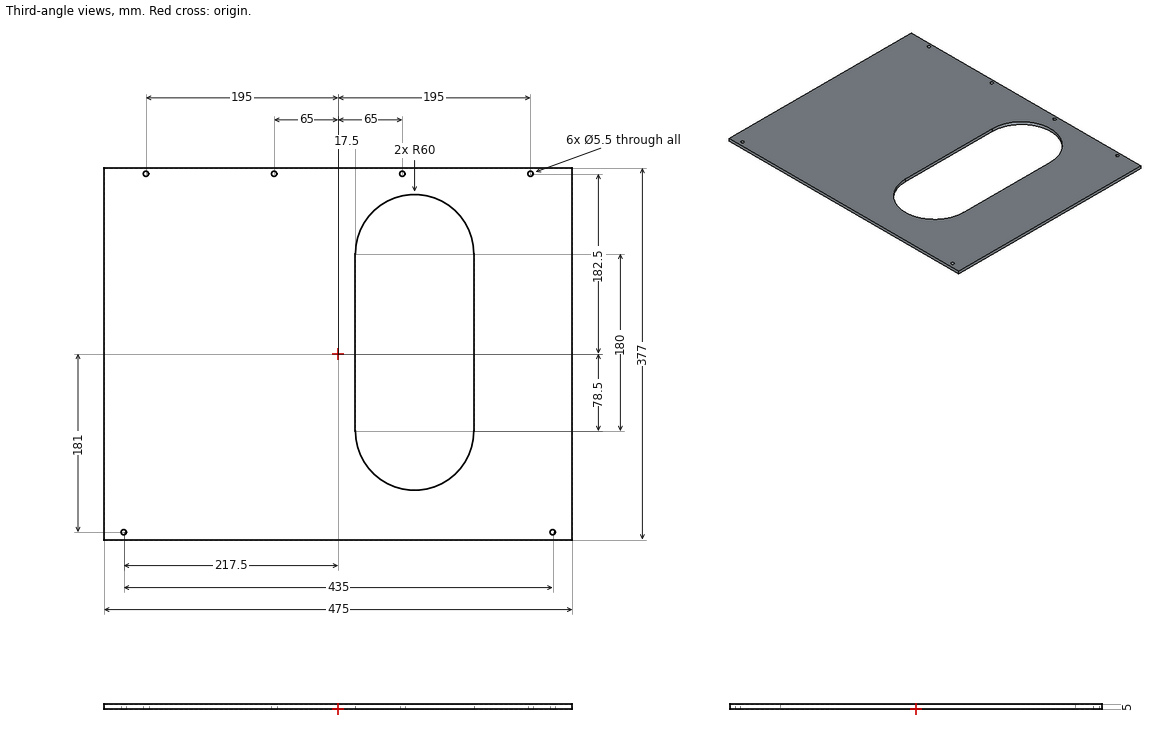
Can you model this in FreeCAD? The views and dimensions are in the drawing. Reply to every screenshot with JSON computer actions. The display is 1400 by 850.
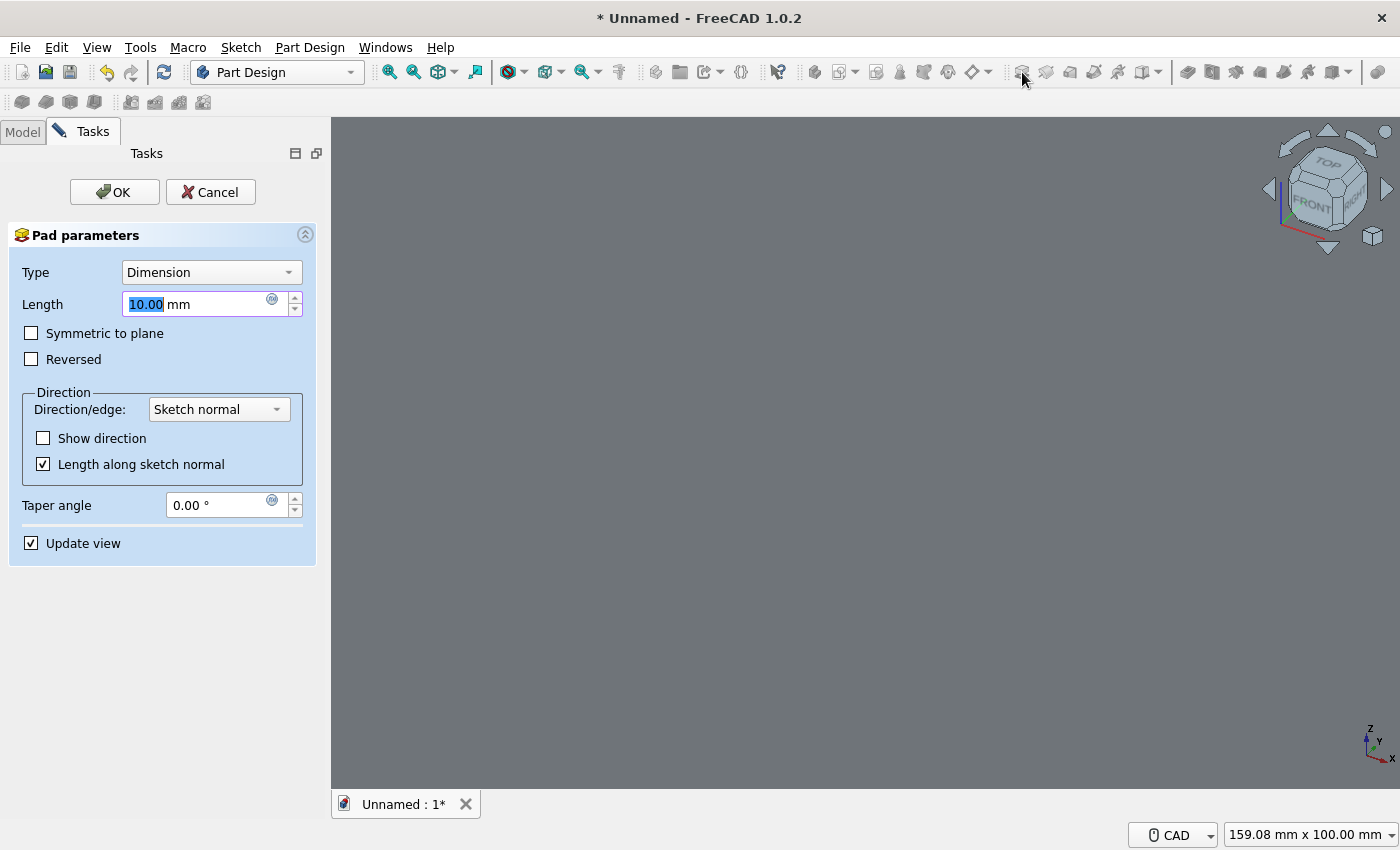
{"action": "type", "text": "5"}
{"action": "key", "text": "Tab"}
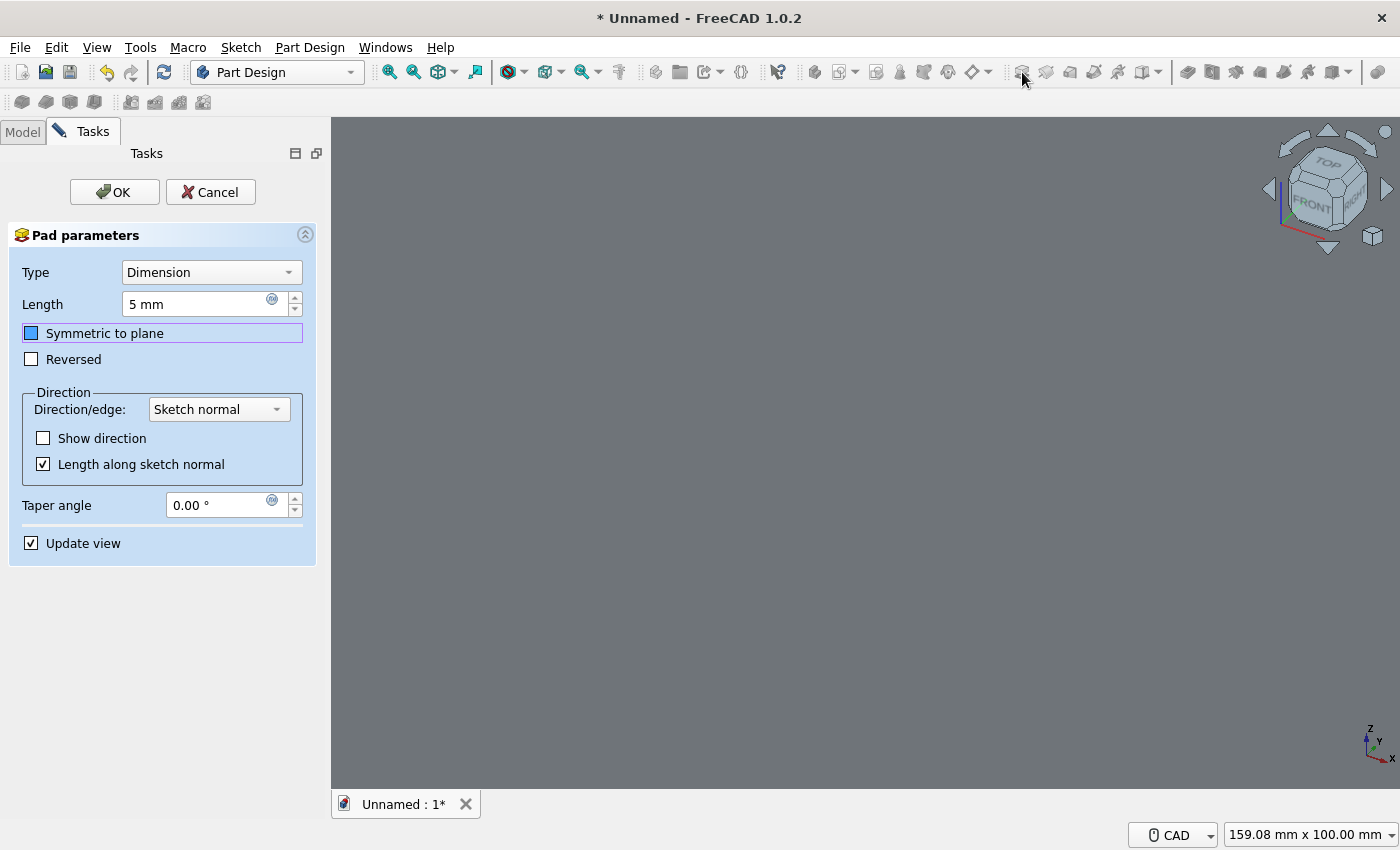
{"action": "left_click", "coordinate": [115, 192]}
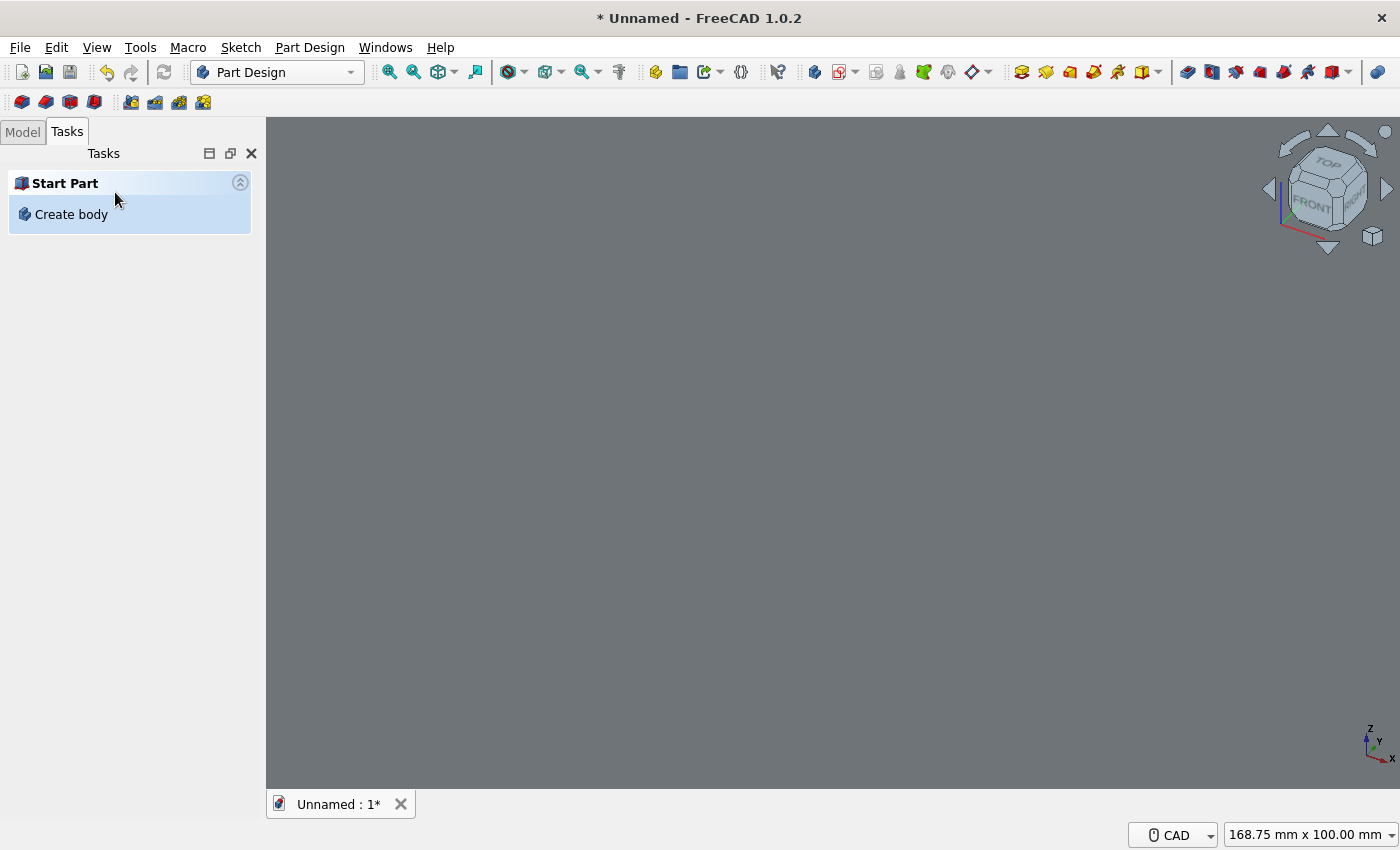
{"action": "key", "text": "v f"}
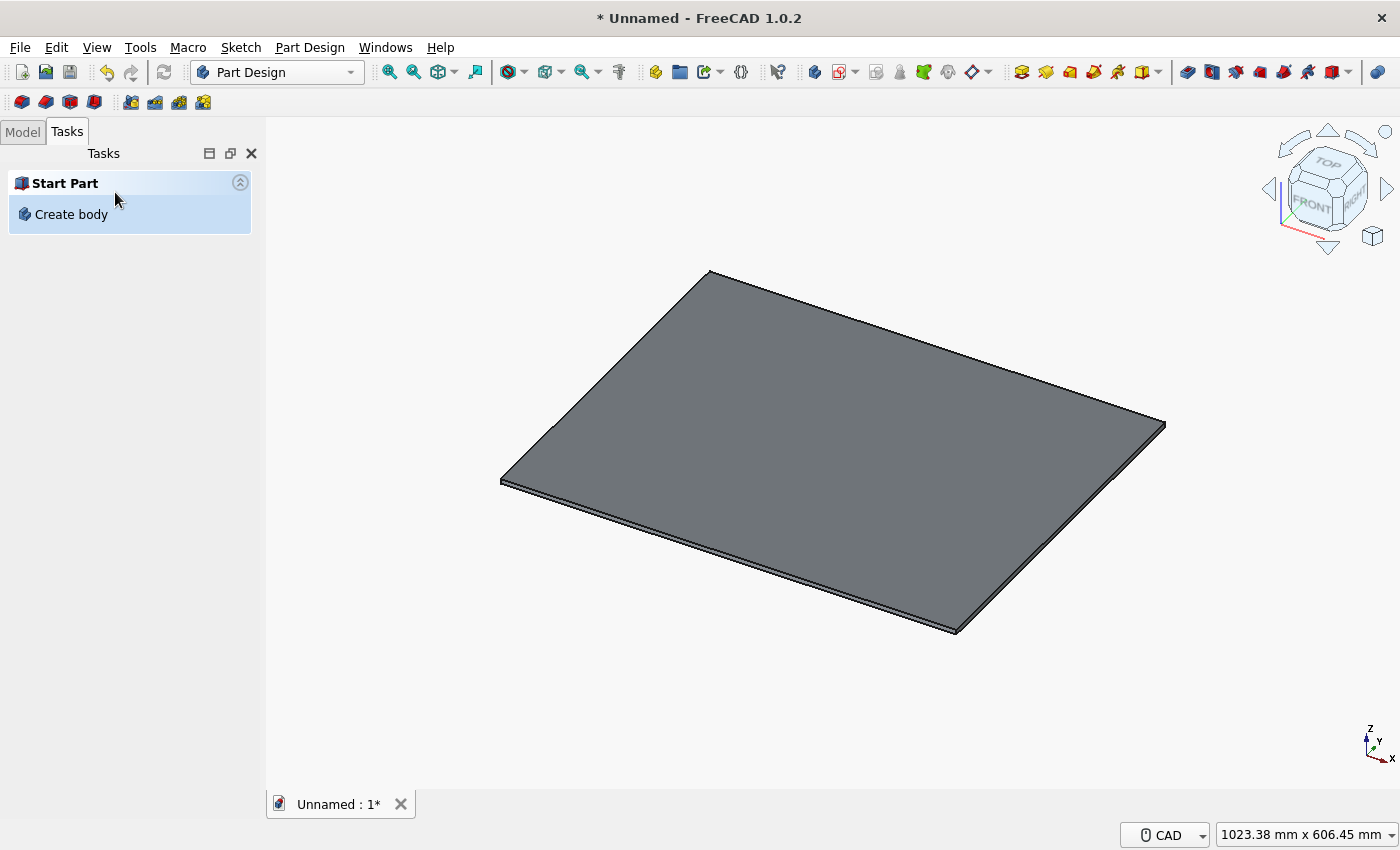
{"action": "key", "text": "5"}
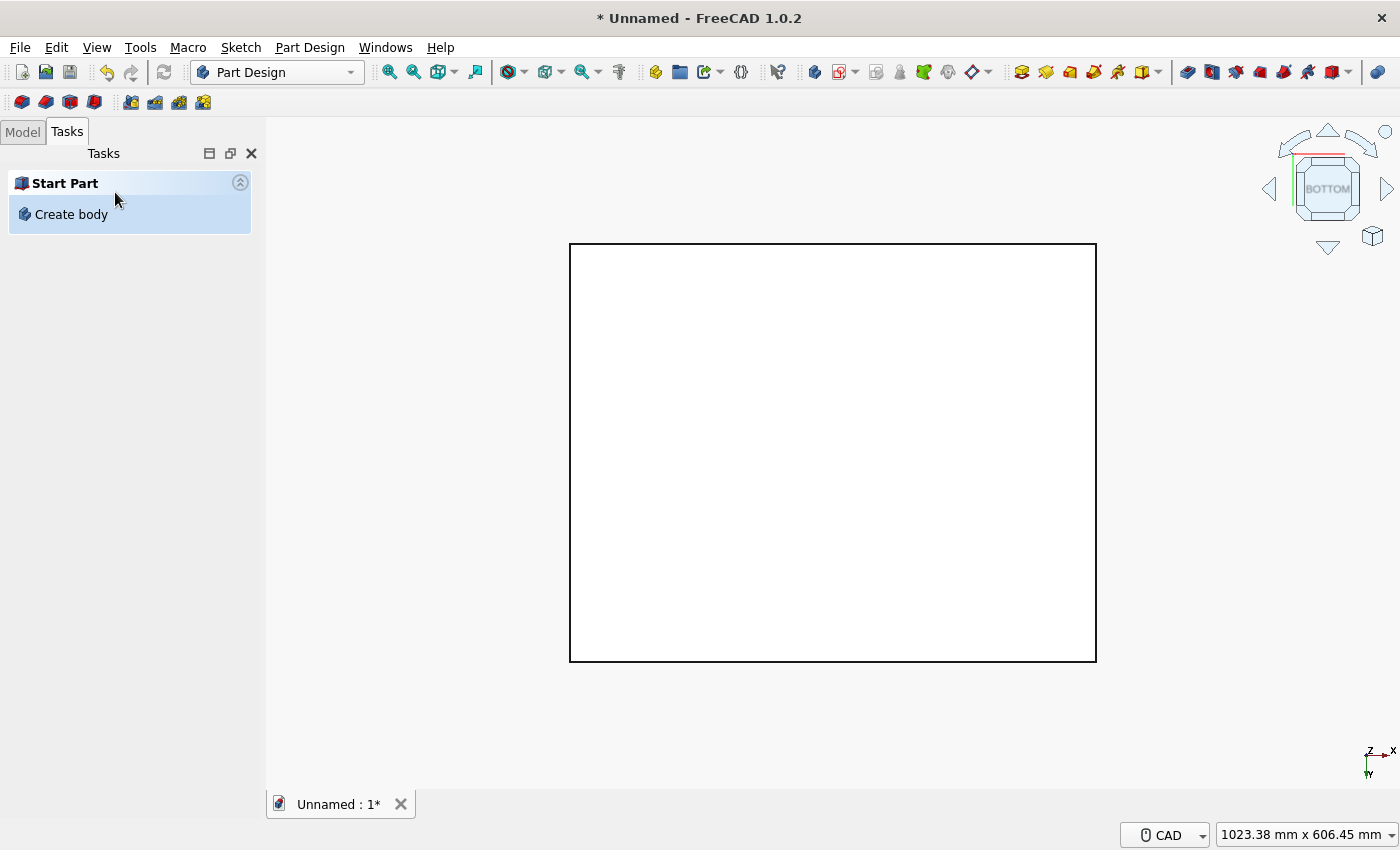
{"action": "left_click", "coordinate": [833, 452]}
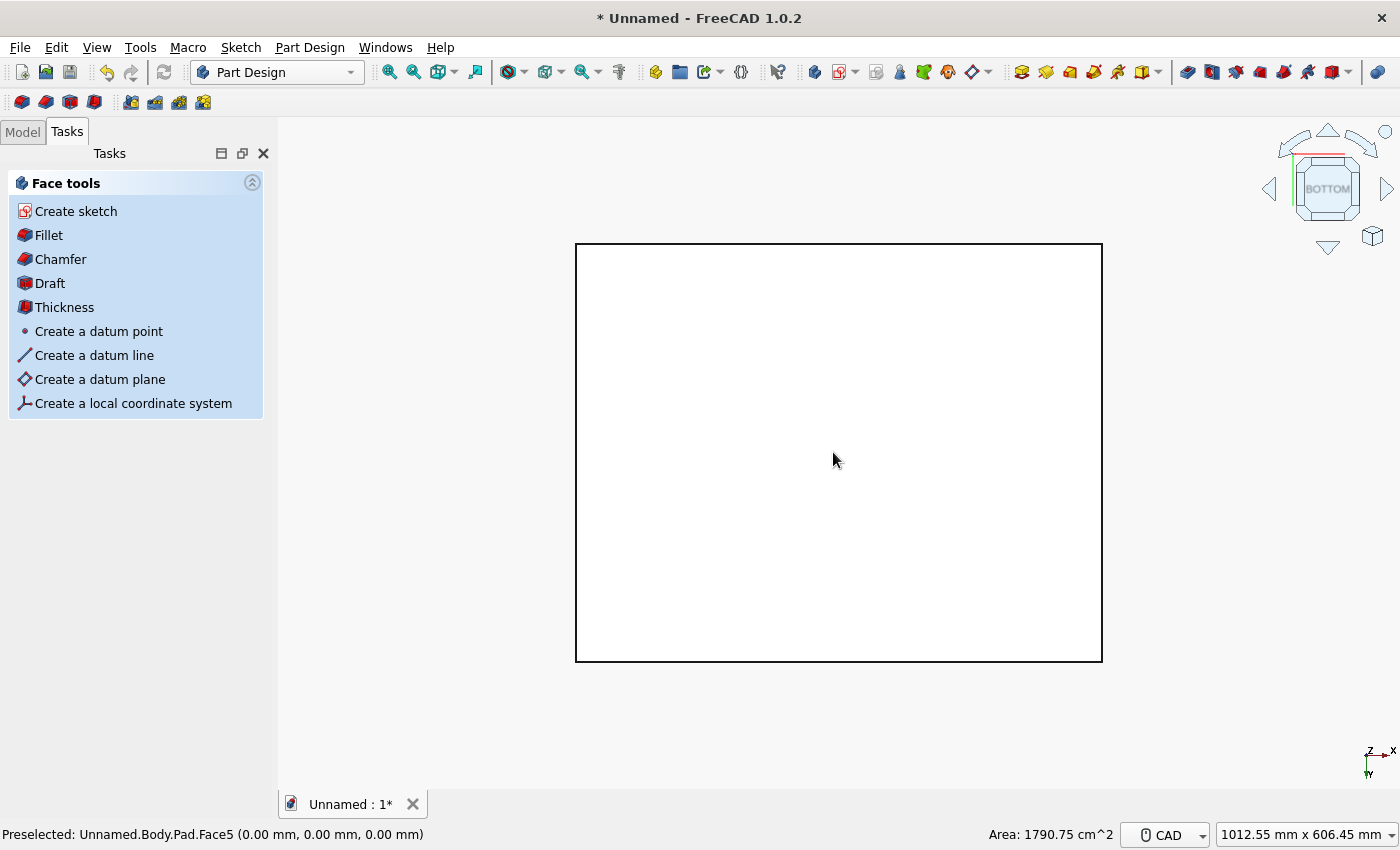
{"action": "left_click", "coordinate": [840, 72]}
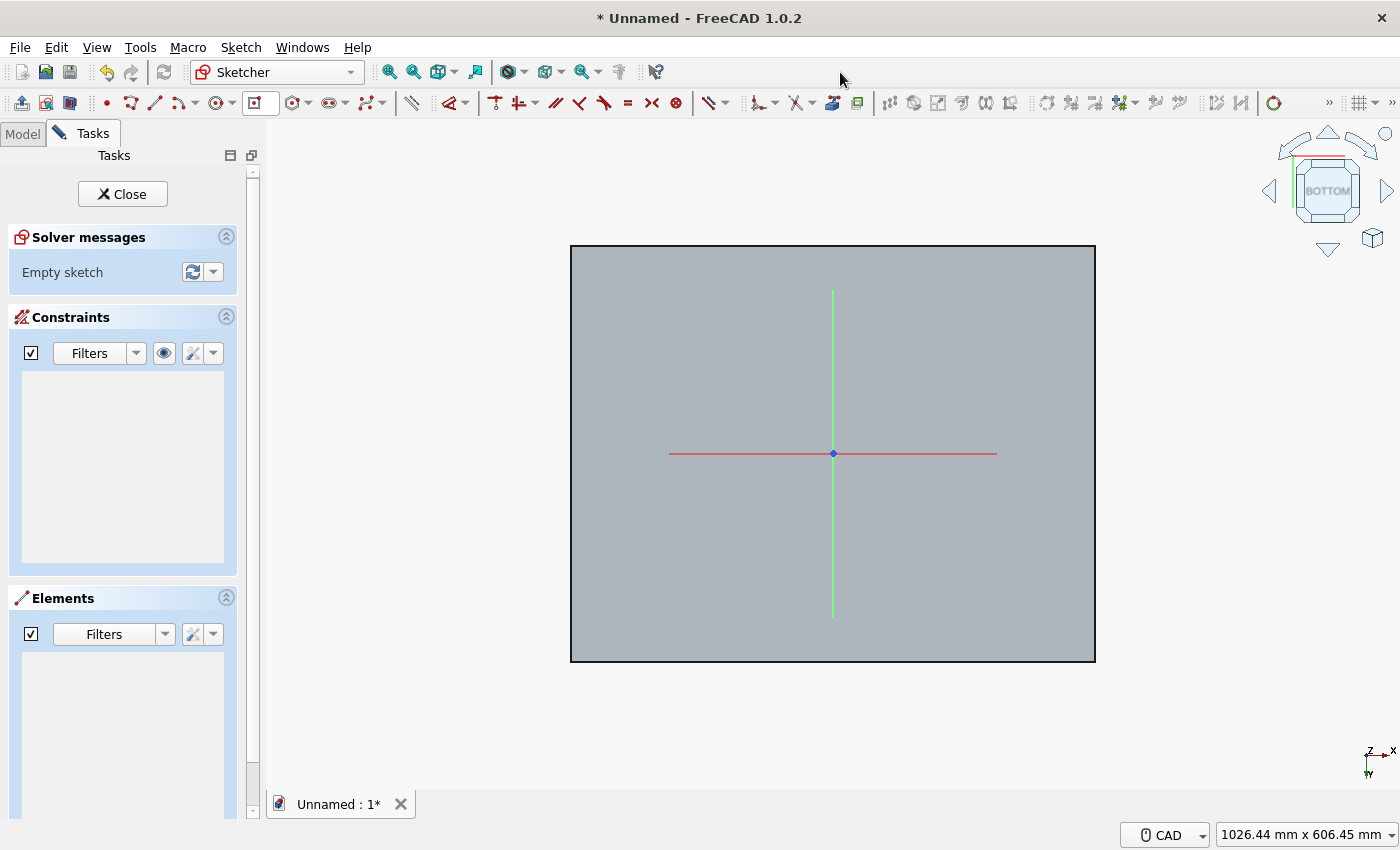
{"action": "key", "text": "g c"}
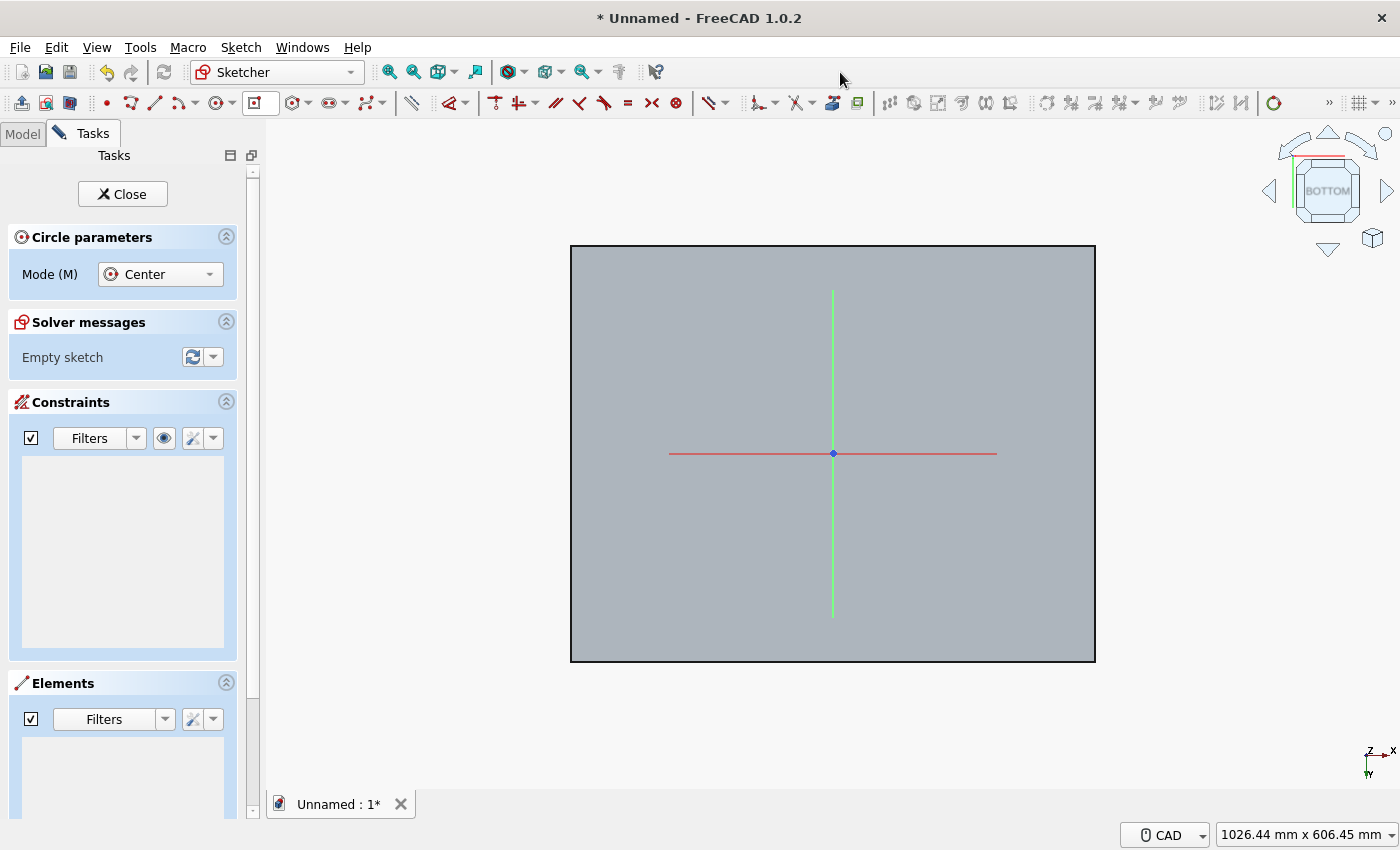
{"action": "scroll", "coordinate": [1048, 656], "scroll_direction": "up", "scroll_amount": 11}